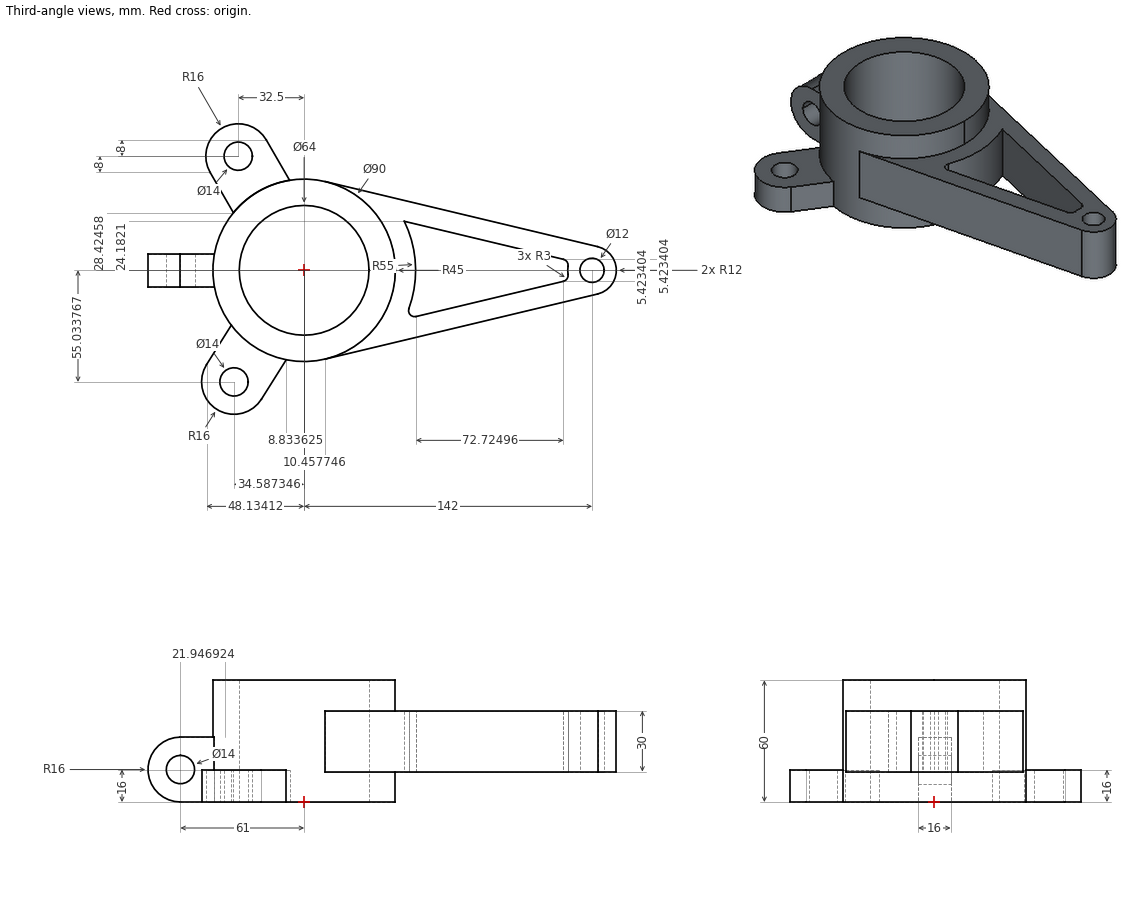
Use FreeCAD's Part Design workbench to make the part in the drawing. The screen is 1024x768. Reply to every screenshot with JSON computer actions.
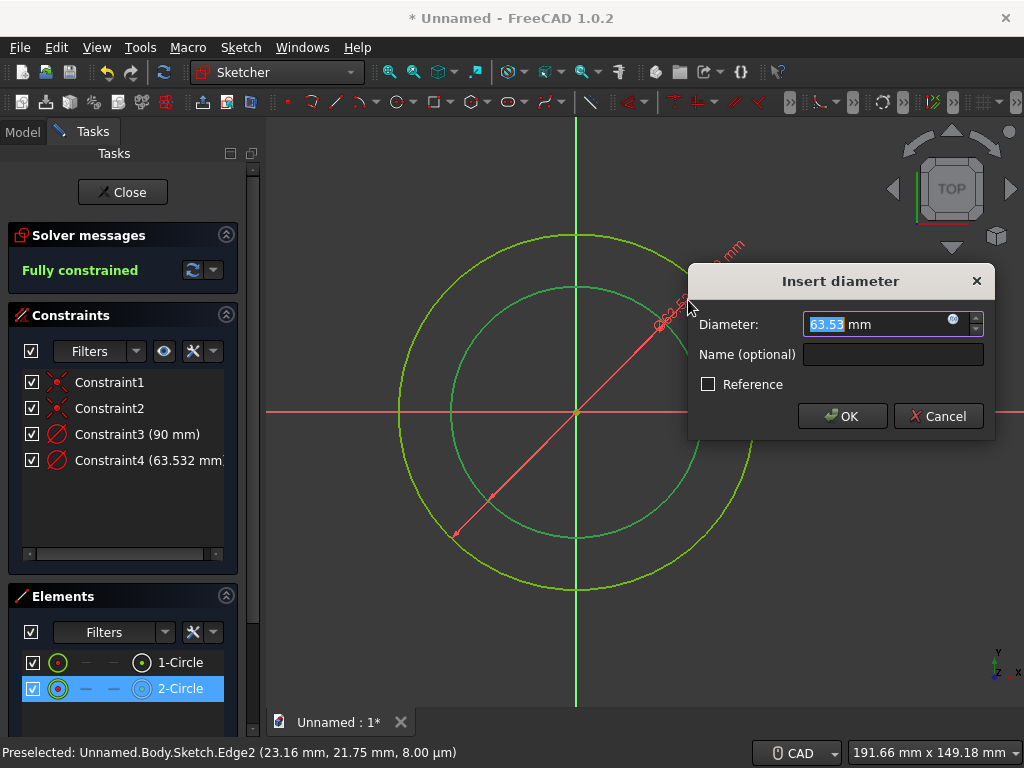
{"action": "type", "text": "64"}
{"action": "key", "text": "Return"}
{"action": "key", "text": "Escape"}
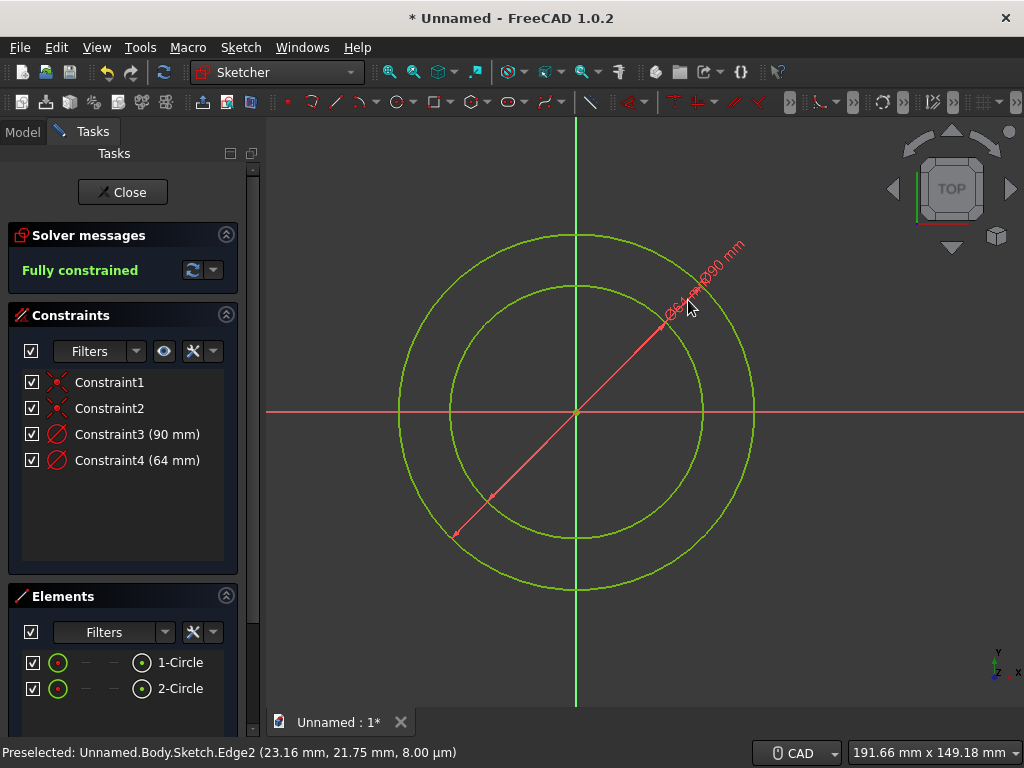
{"action": "left_click", "coordinate": [123, 192]}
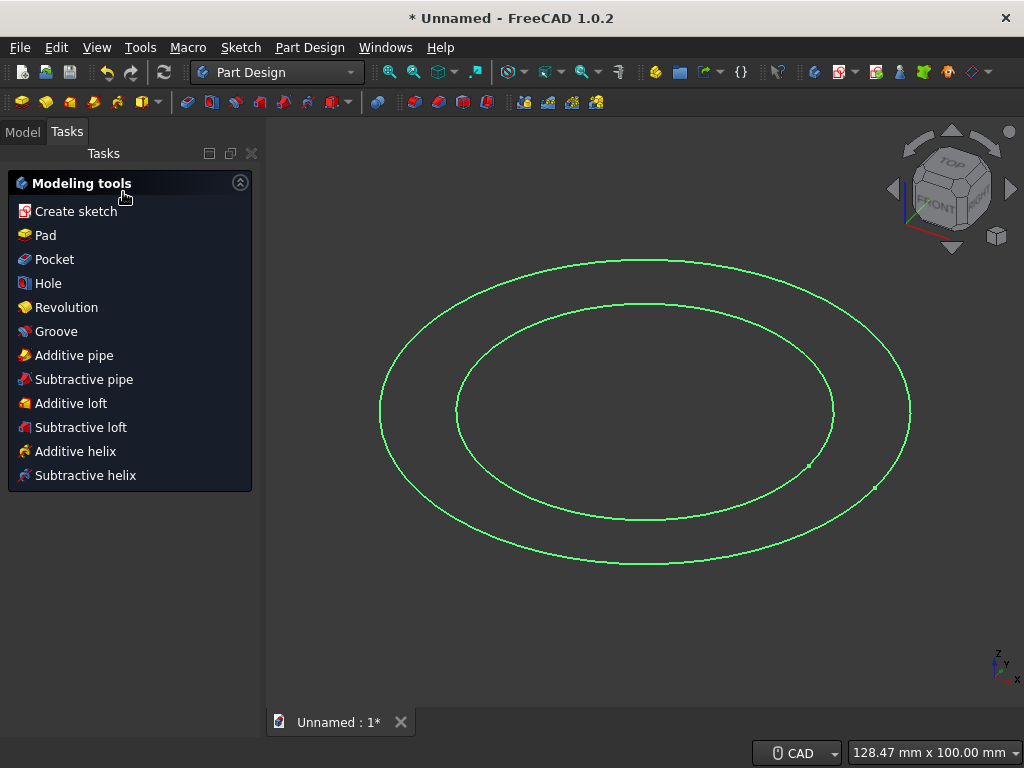
{"action": "left_click", "coordinate": [22, 102]}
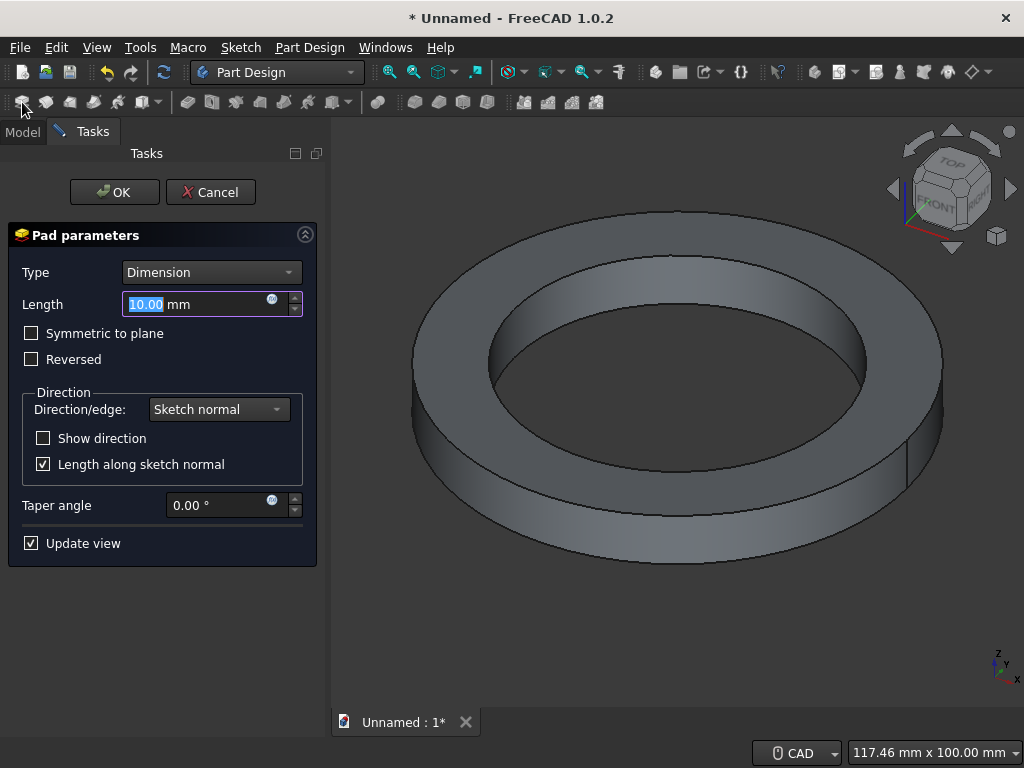
{"action": "type", "text": "60"}
{"action": "key", "text": "Tab"}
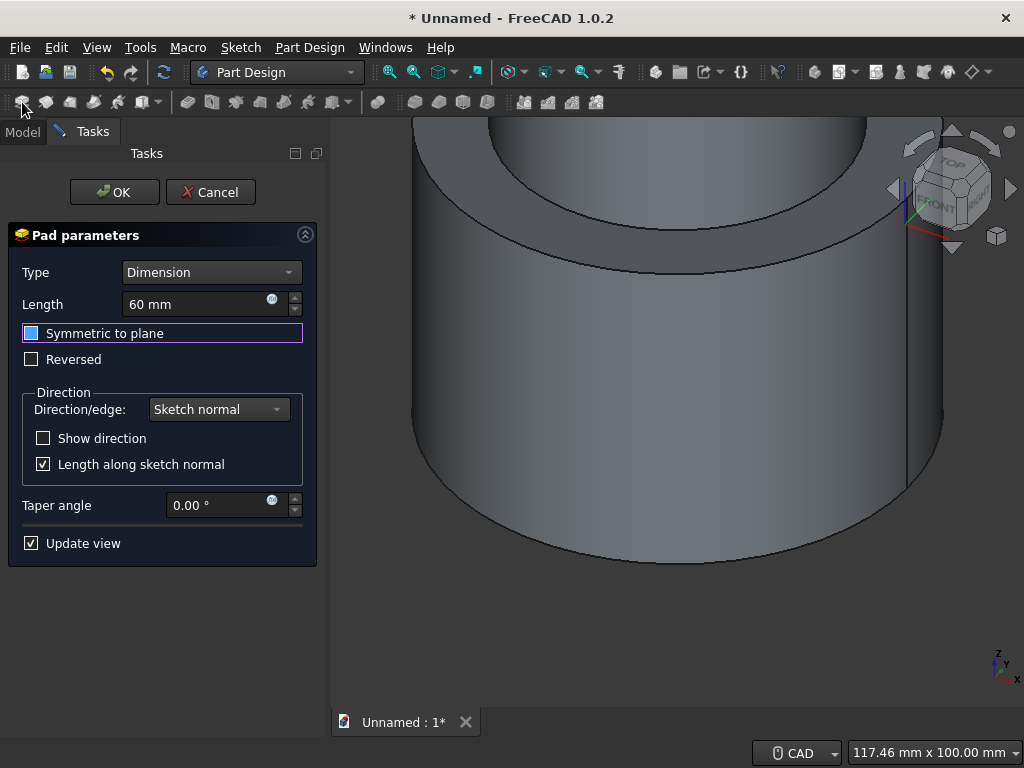
{"action": "left_click", "coordinate": [115, 192]}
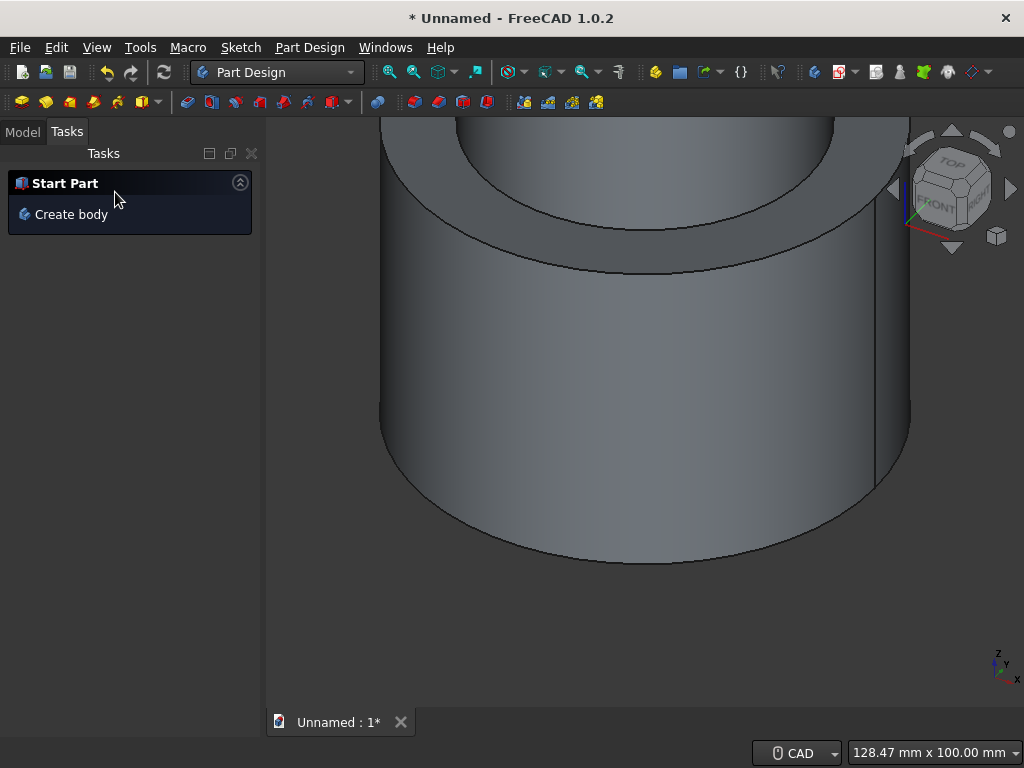
{"action": "key", "text": "v f"}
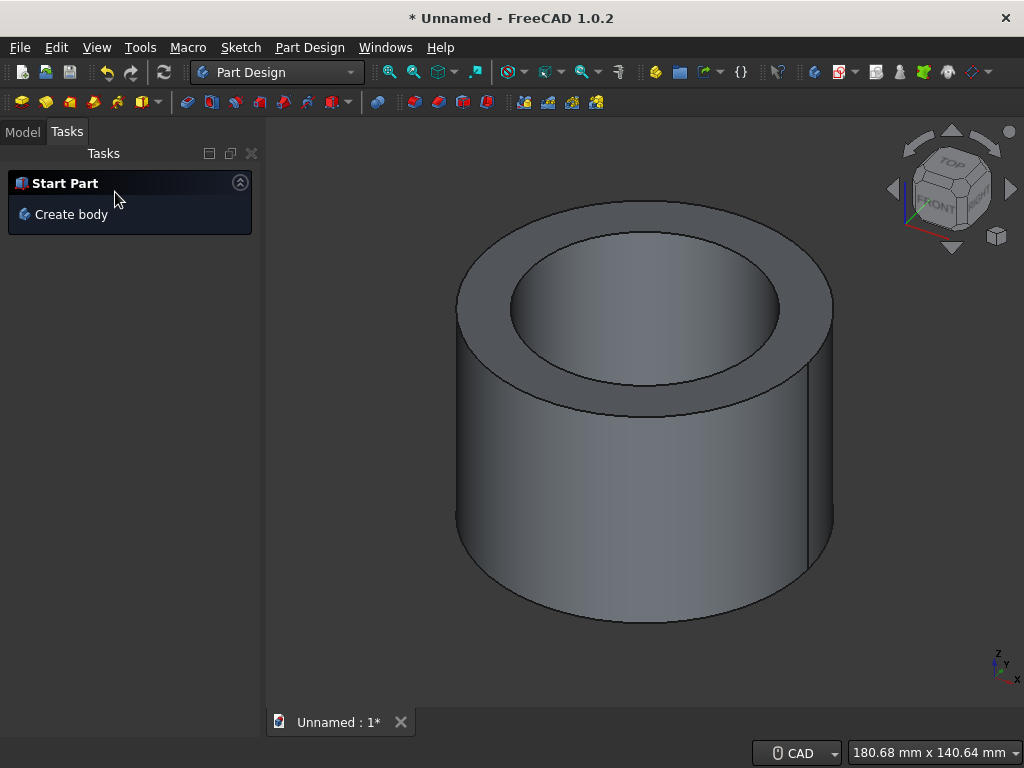
{"action": "left_click", "coordinate": [23, 131]}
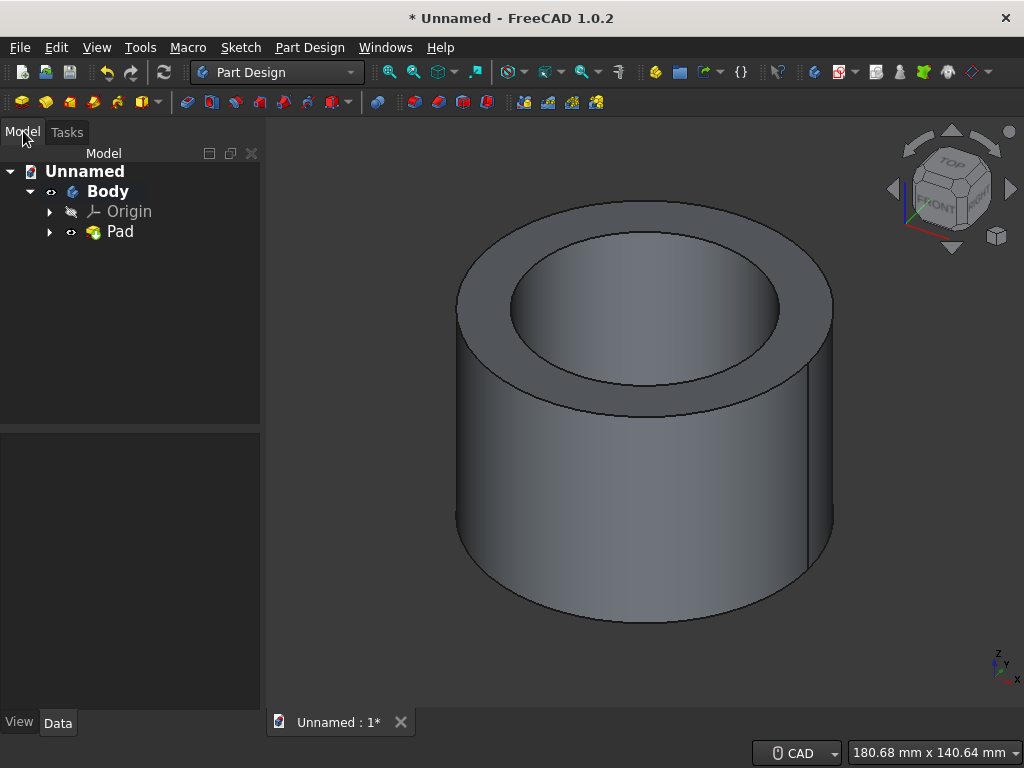
{"action": "left_click", "coordinate": [50, 212]}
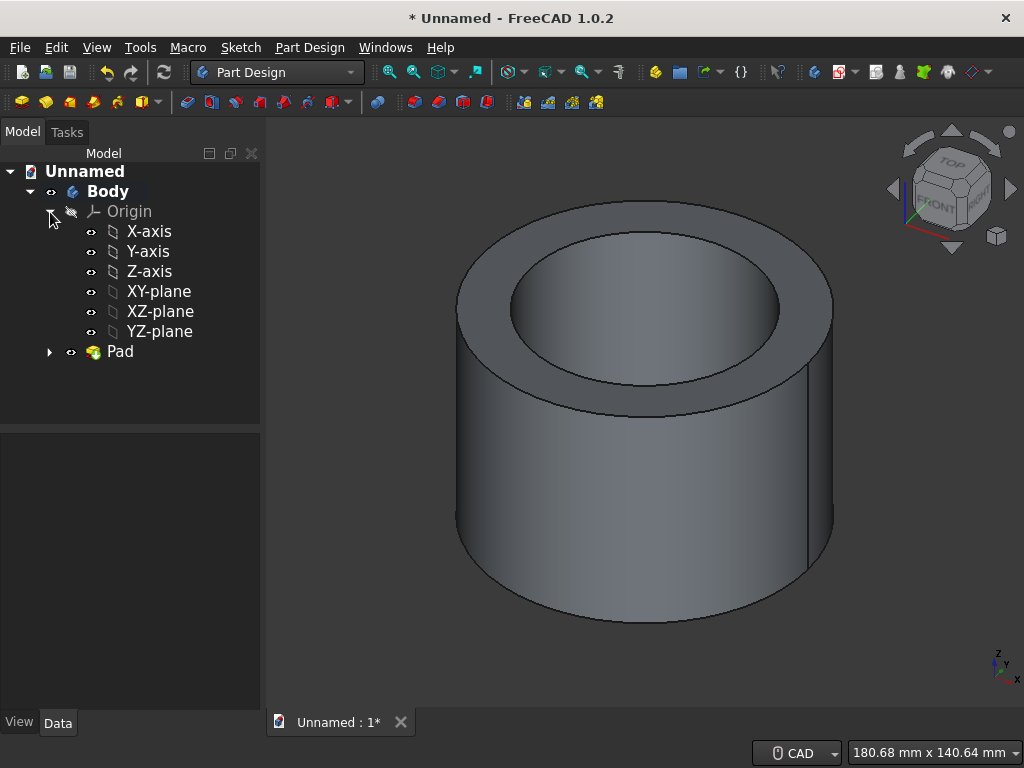
{"action": "left_click", "coordinate": [136, 292]}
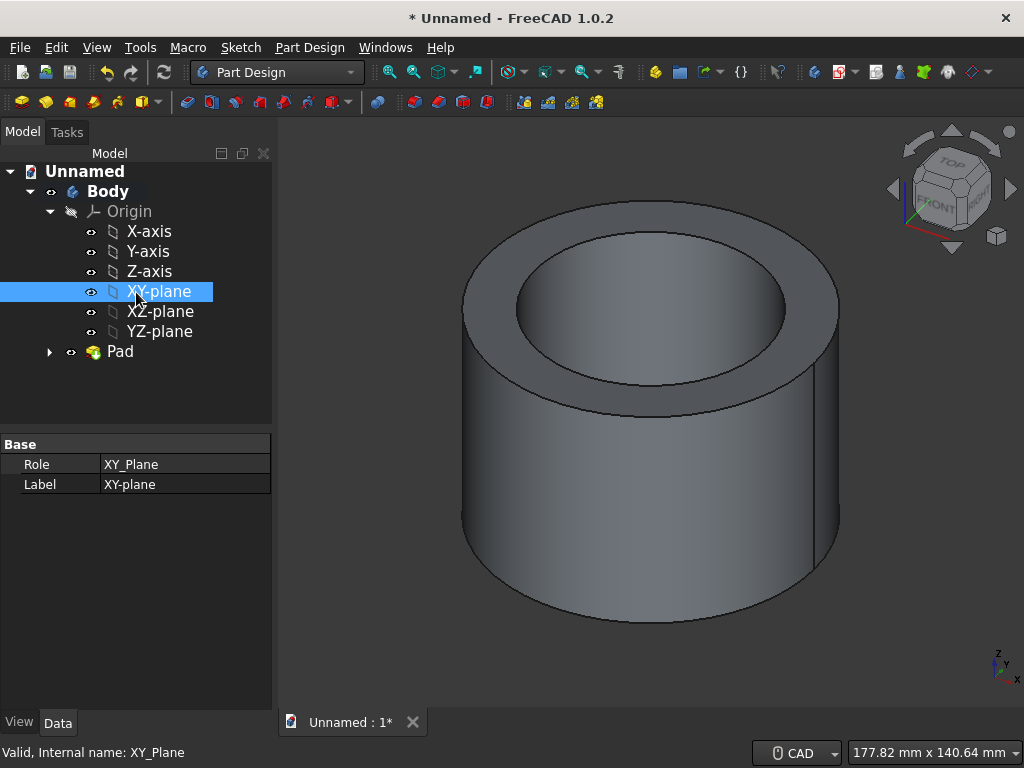
{"action": "left_click", "coordinate": [972, 72]}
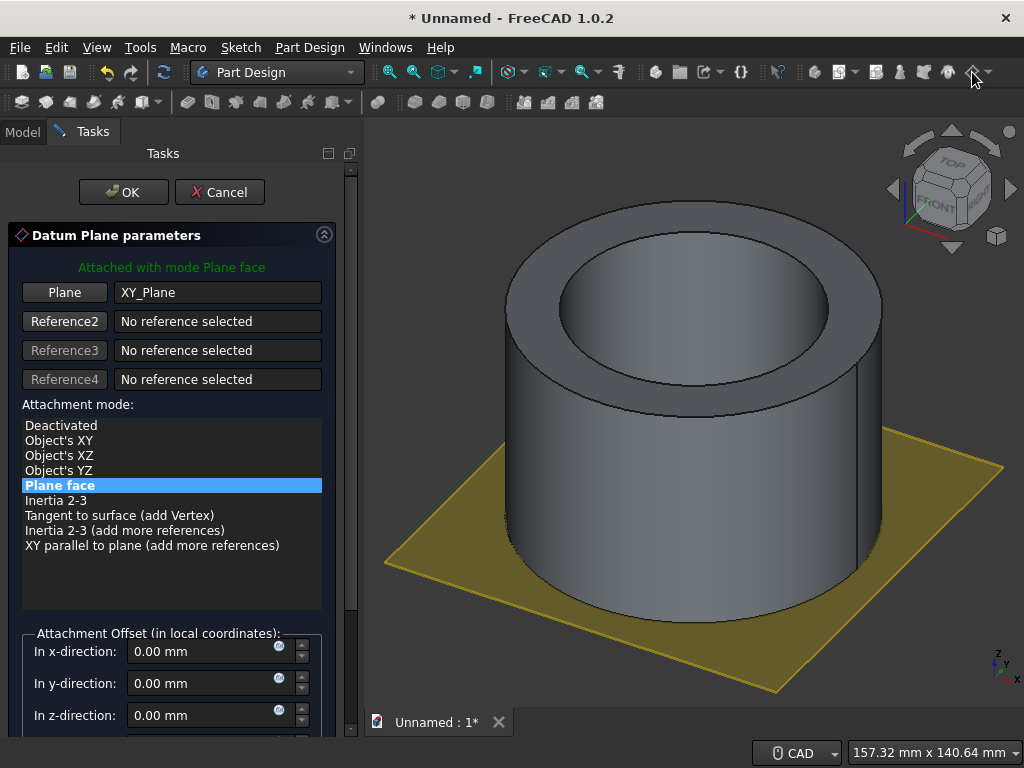
{"action": "triple_click", "coordinate": [210, 715]}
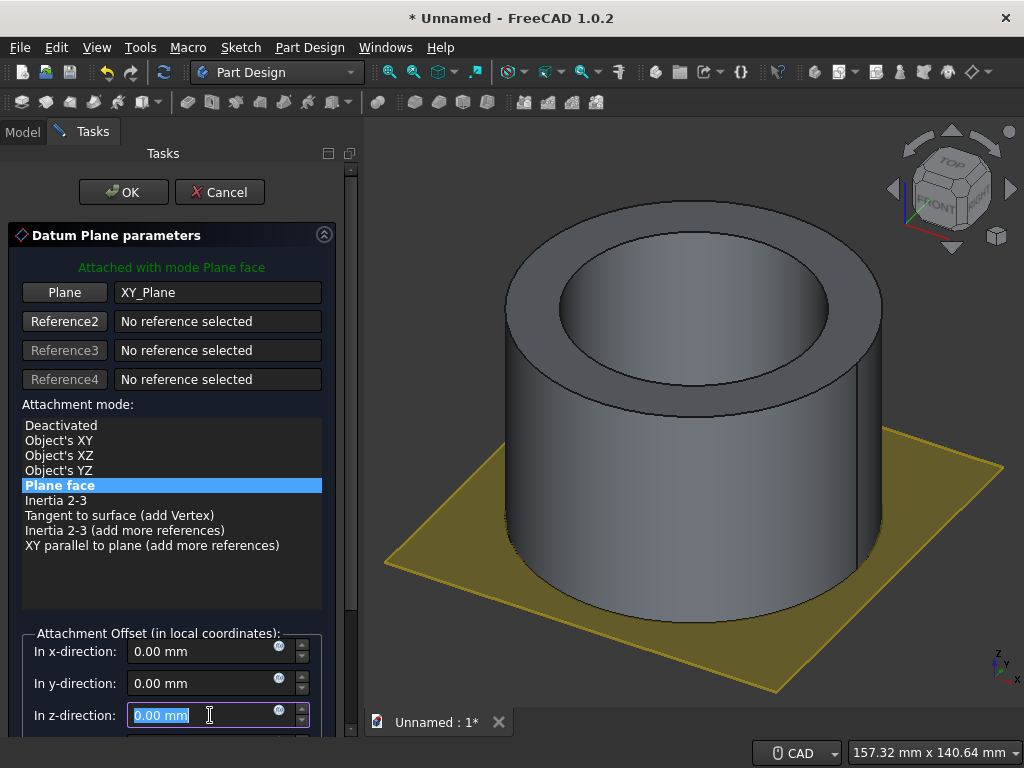
{"action": "type", "text": "30"}
{"action": "key", "text": "Tab"}